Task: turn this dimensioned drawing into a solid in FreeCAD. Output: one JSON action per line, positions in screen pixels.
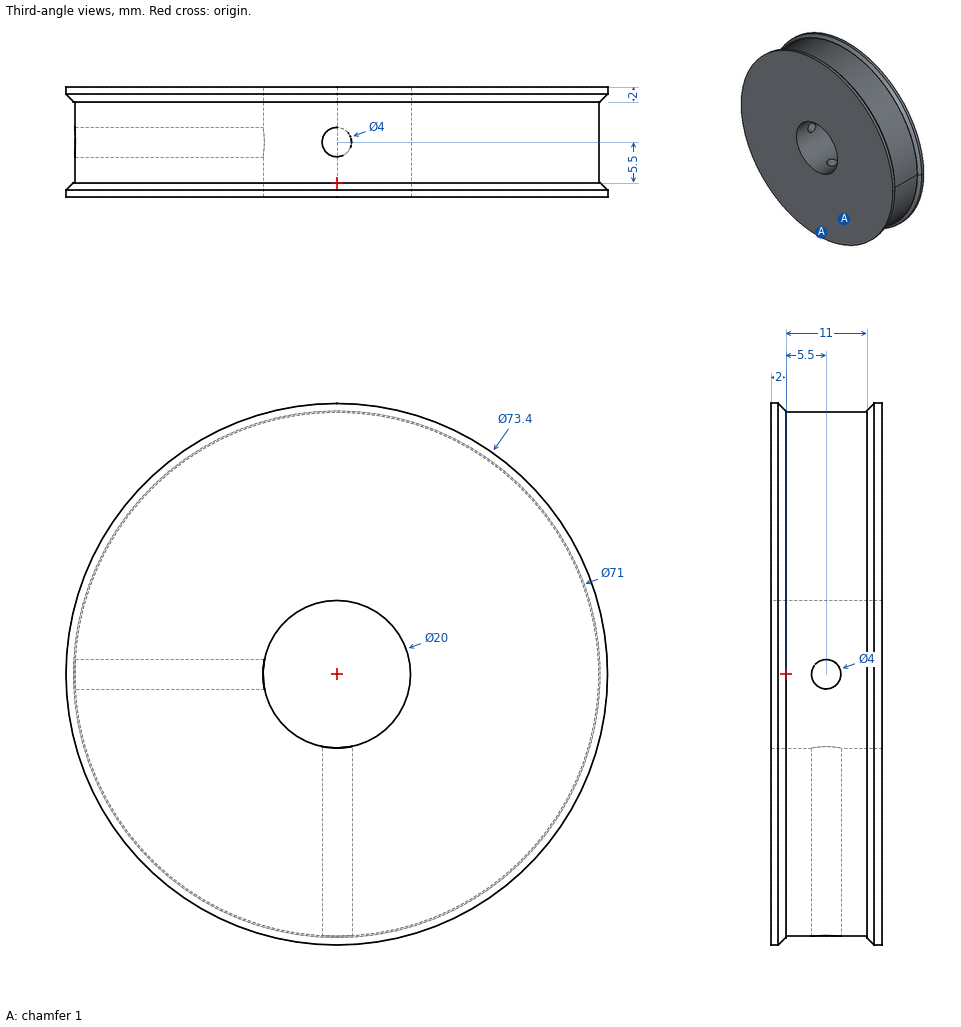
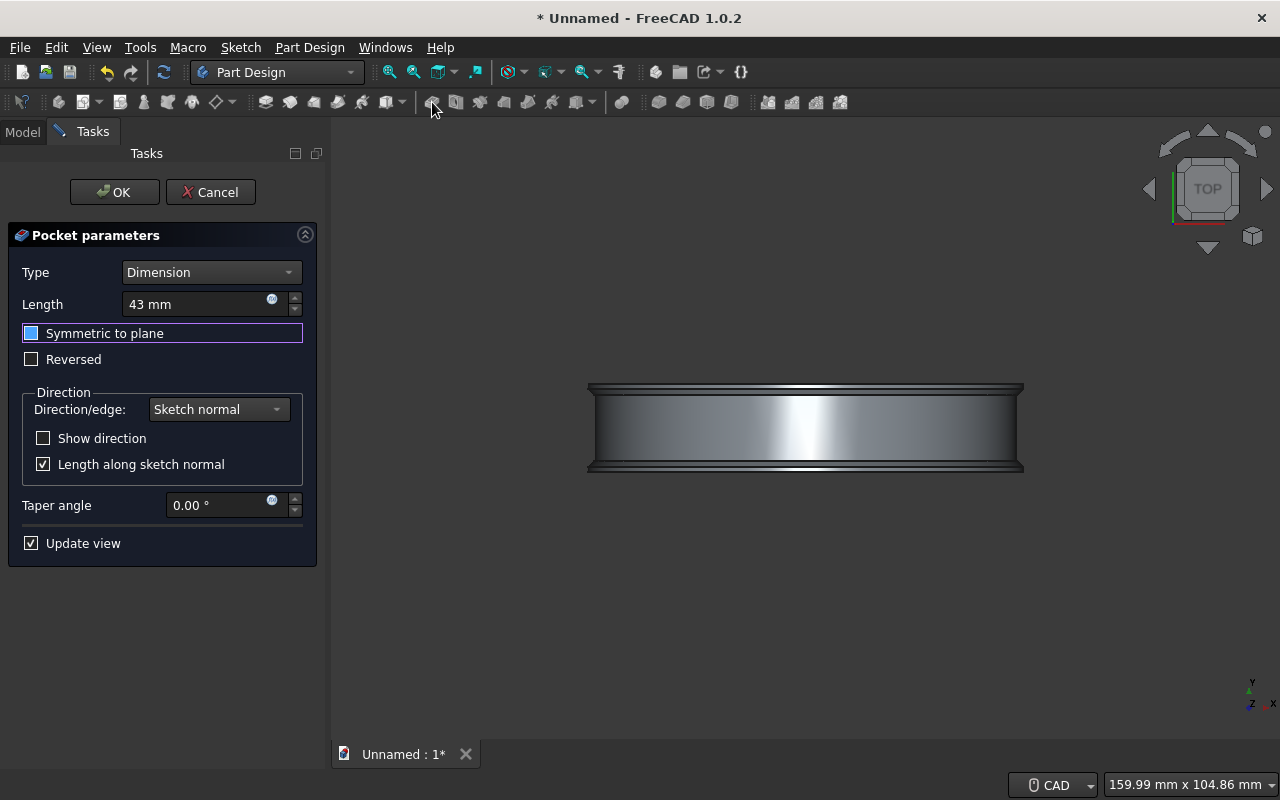
{"action": "left_click", "coordinate": [115, 192]}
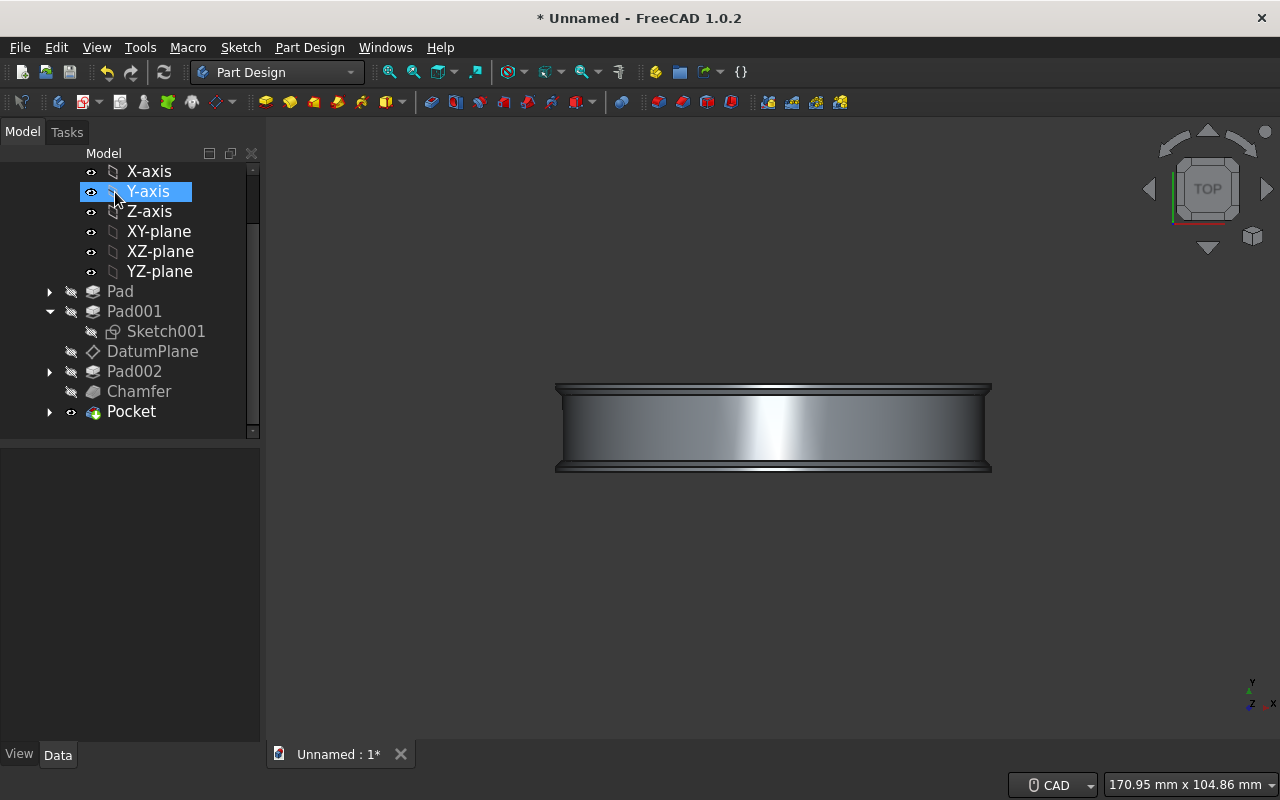
{"action": "left_click", "coordinate": [390, 72]}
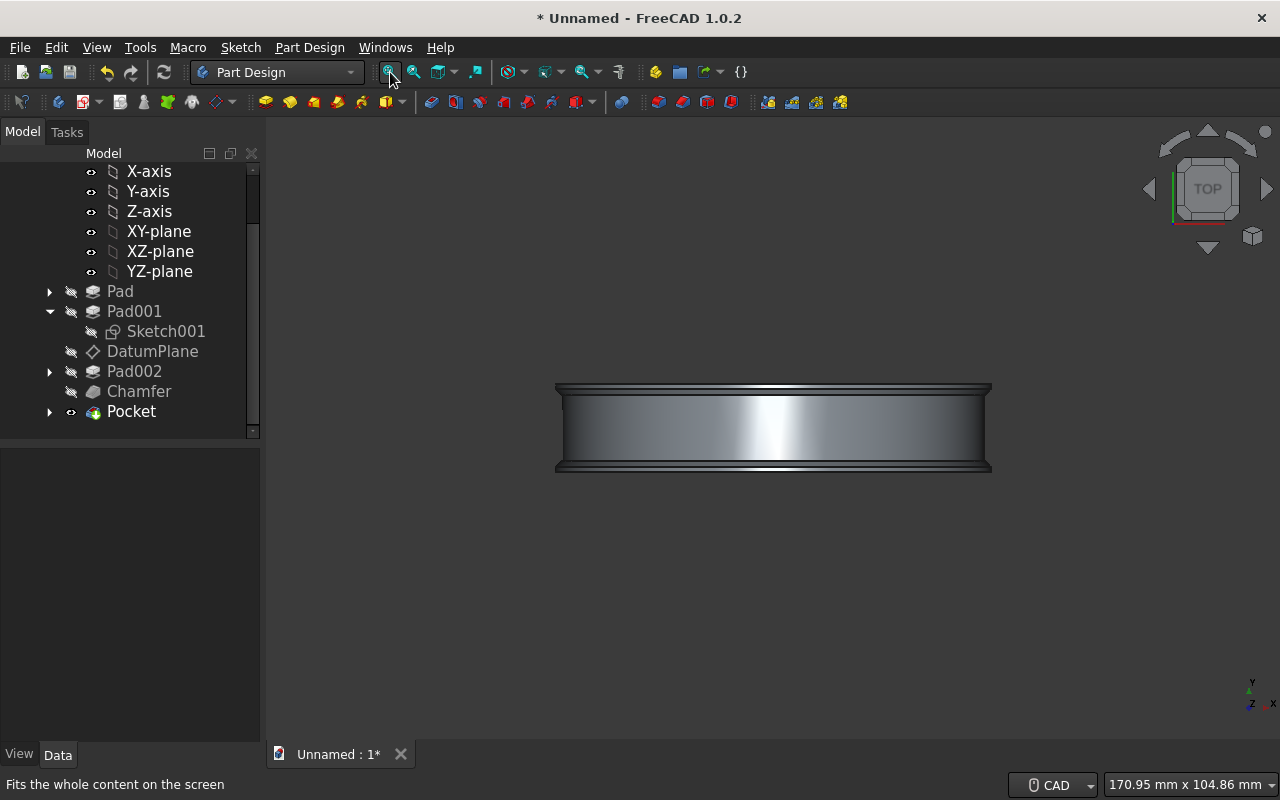
{"action": "left_click", "coordinate": [84, 102]}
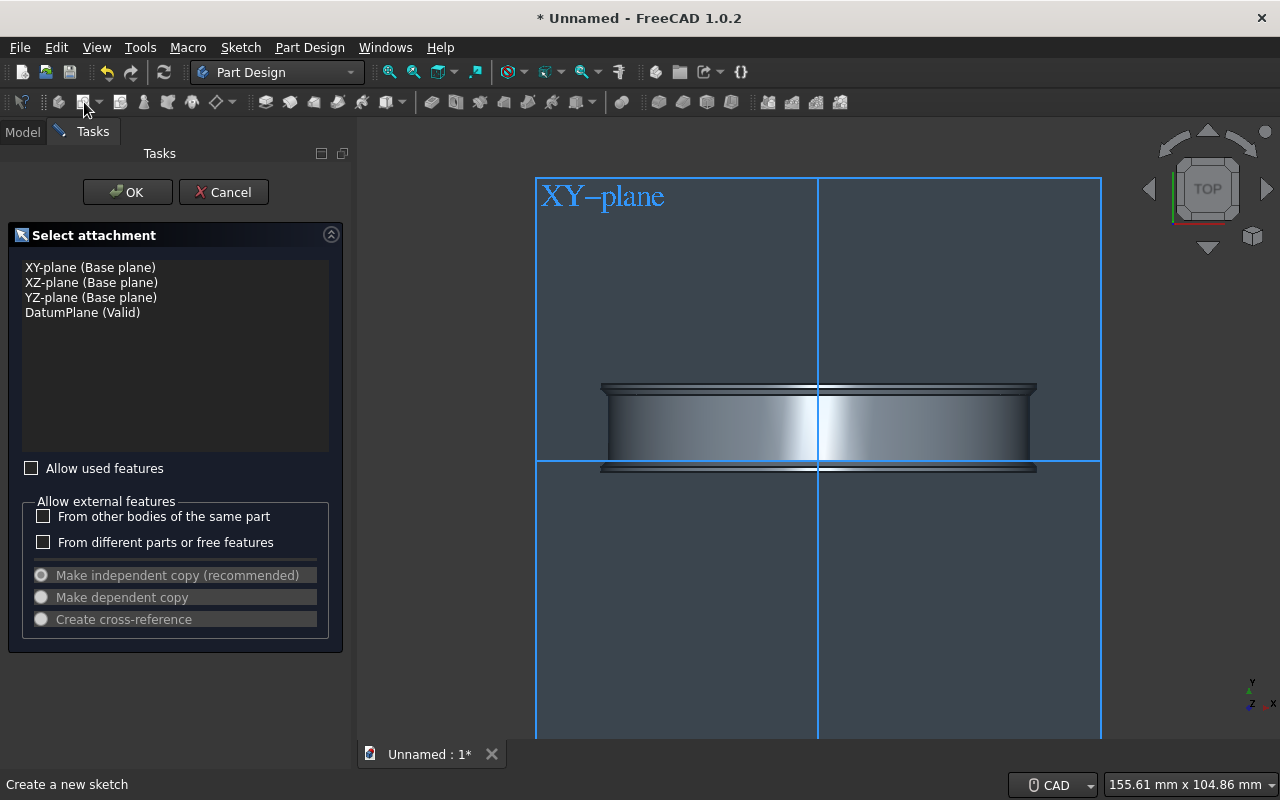
{"action": "left_click", "coordinate": [82, 298]}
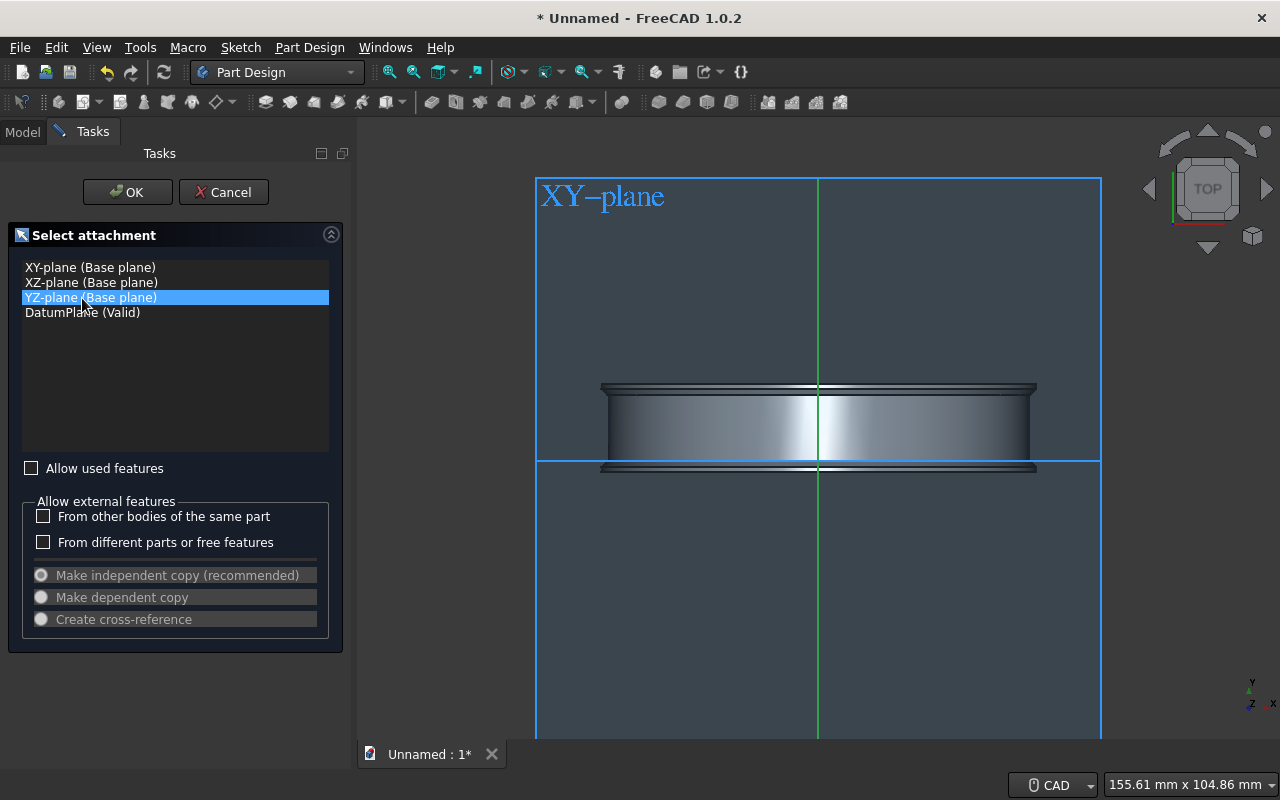
{"action": "left_click", "coordinate": [128, 192]}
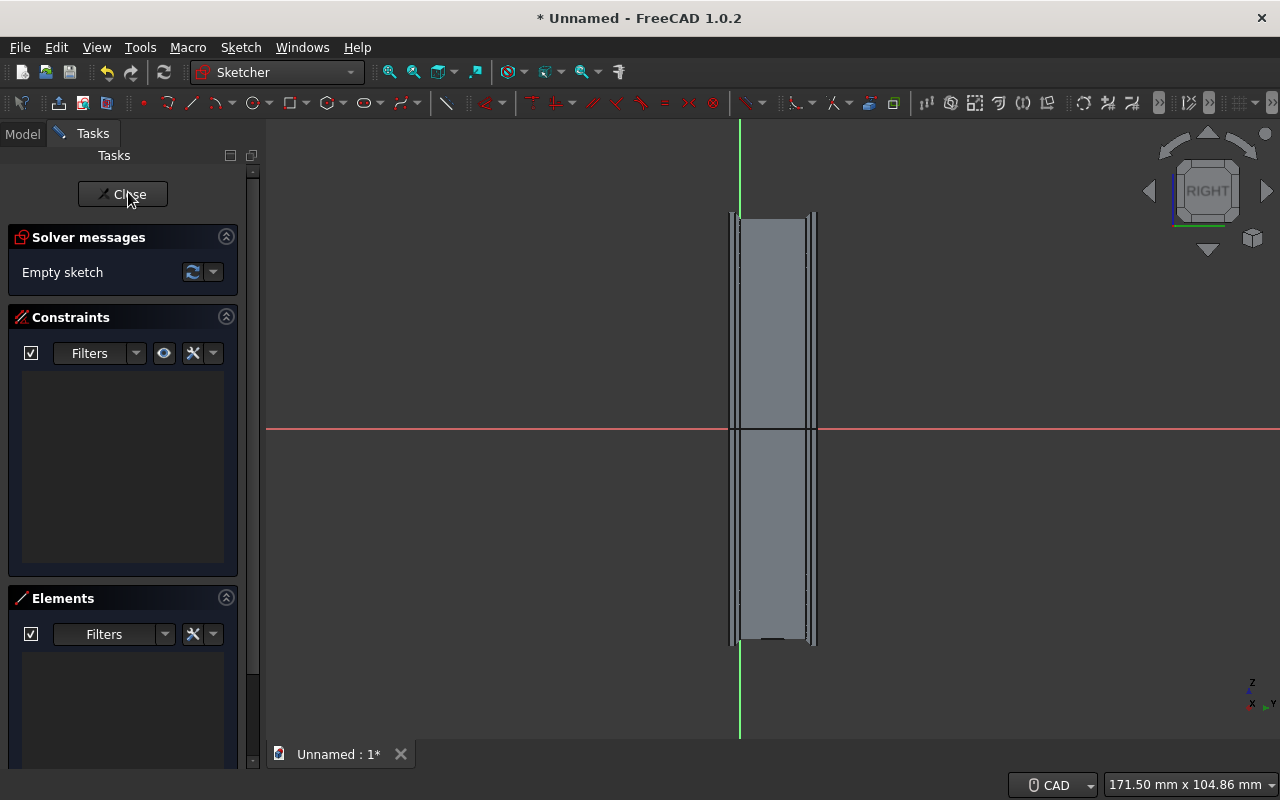
{"action": "left_click", "coordinate": [108, 104]}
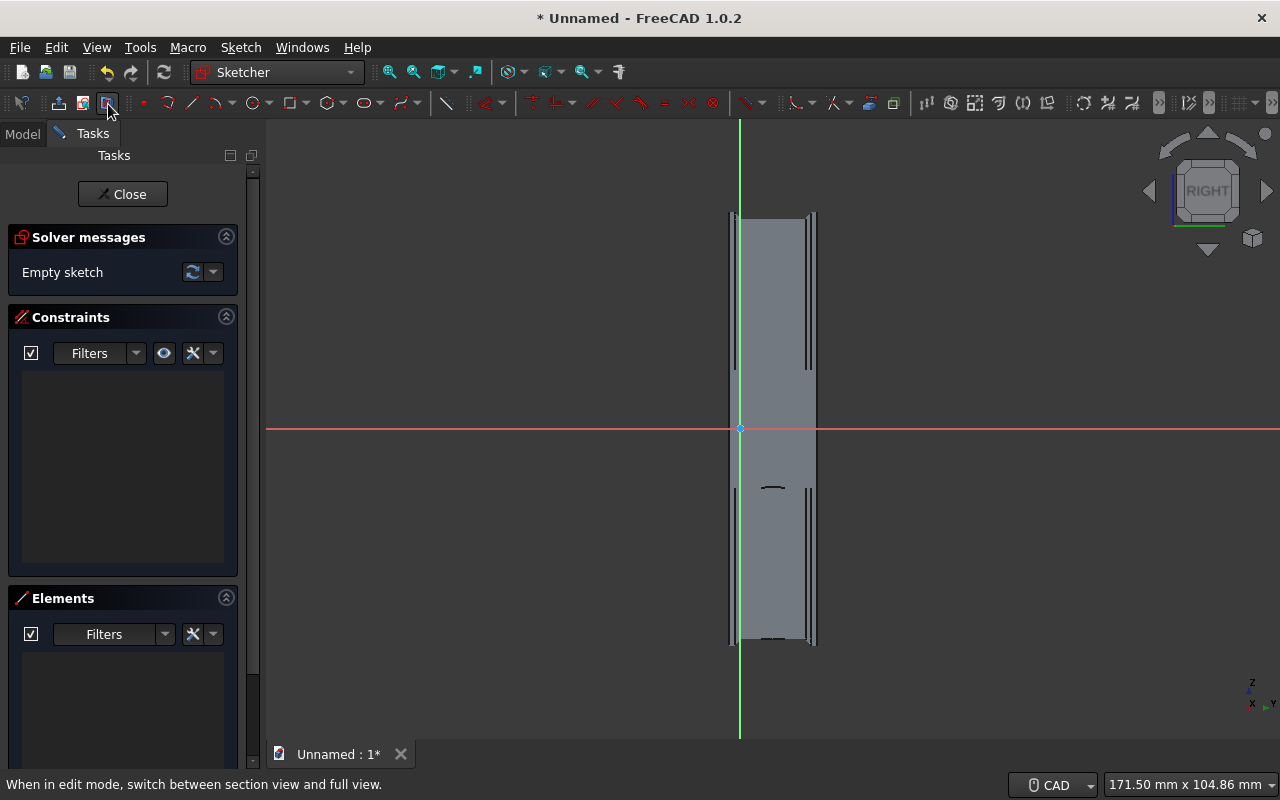
{"action": "scroll", "coordinate": [767, 429], "scroll_direction": "up", "scroll_amount": 13}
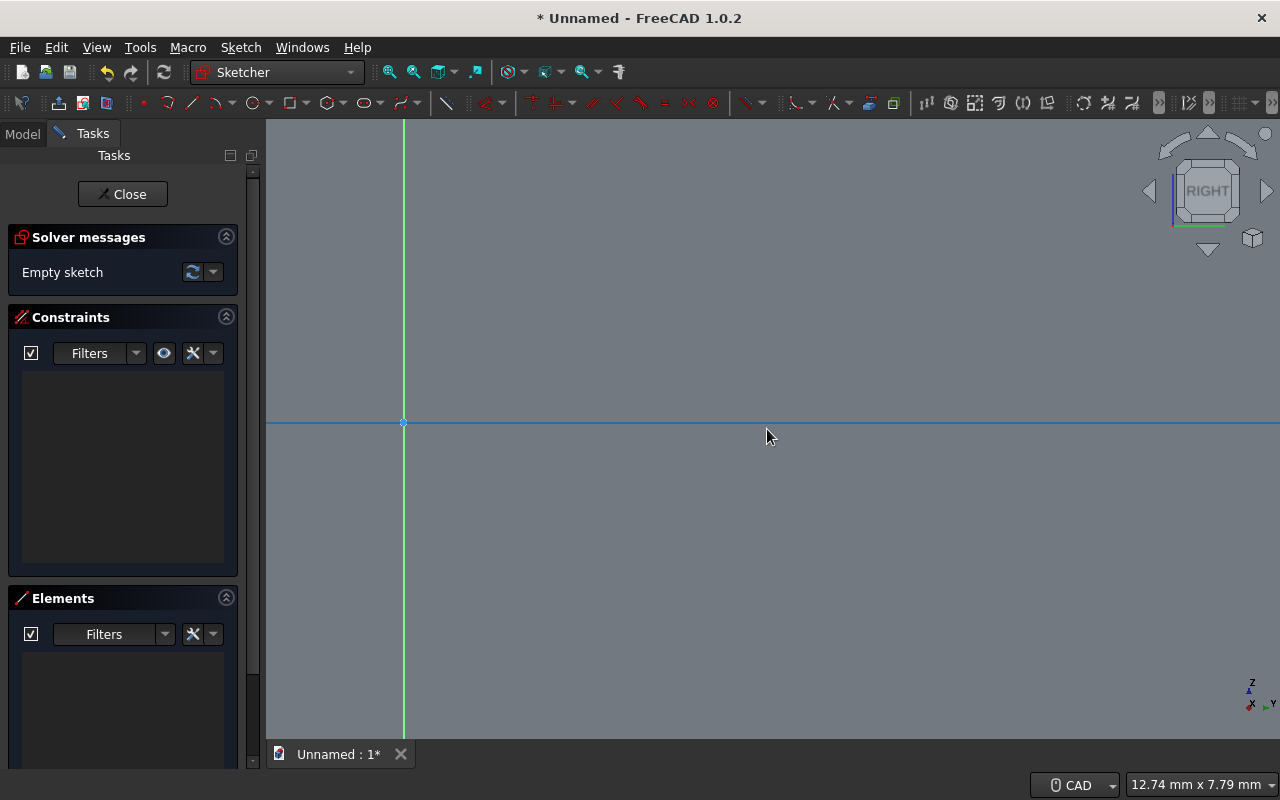
{"action": "left_click", "coordinate": [254, 104]}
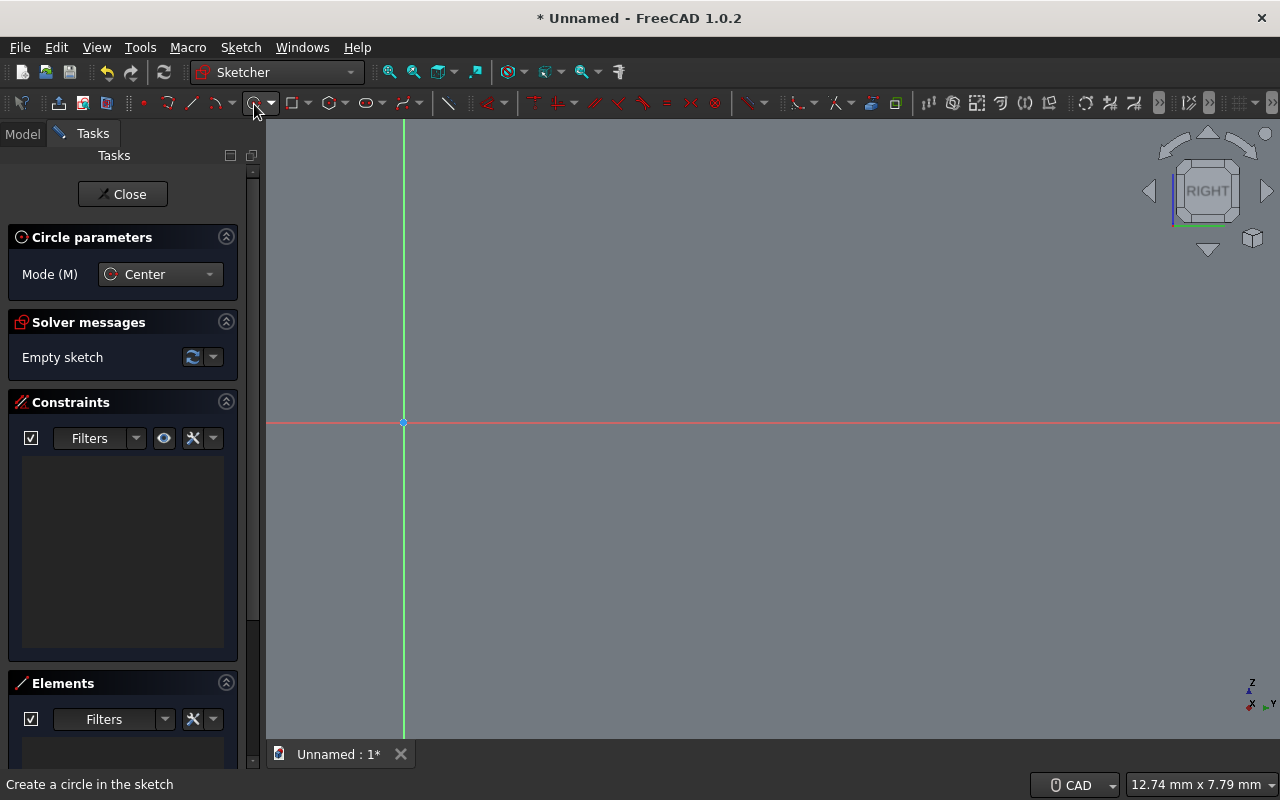
{"action": "left_click", "coordinate": [842, 423]}
{"action": "left_click", "coordinate": [954, 310]}
{"action": "key", "text": "Escape"}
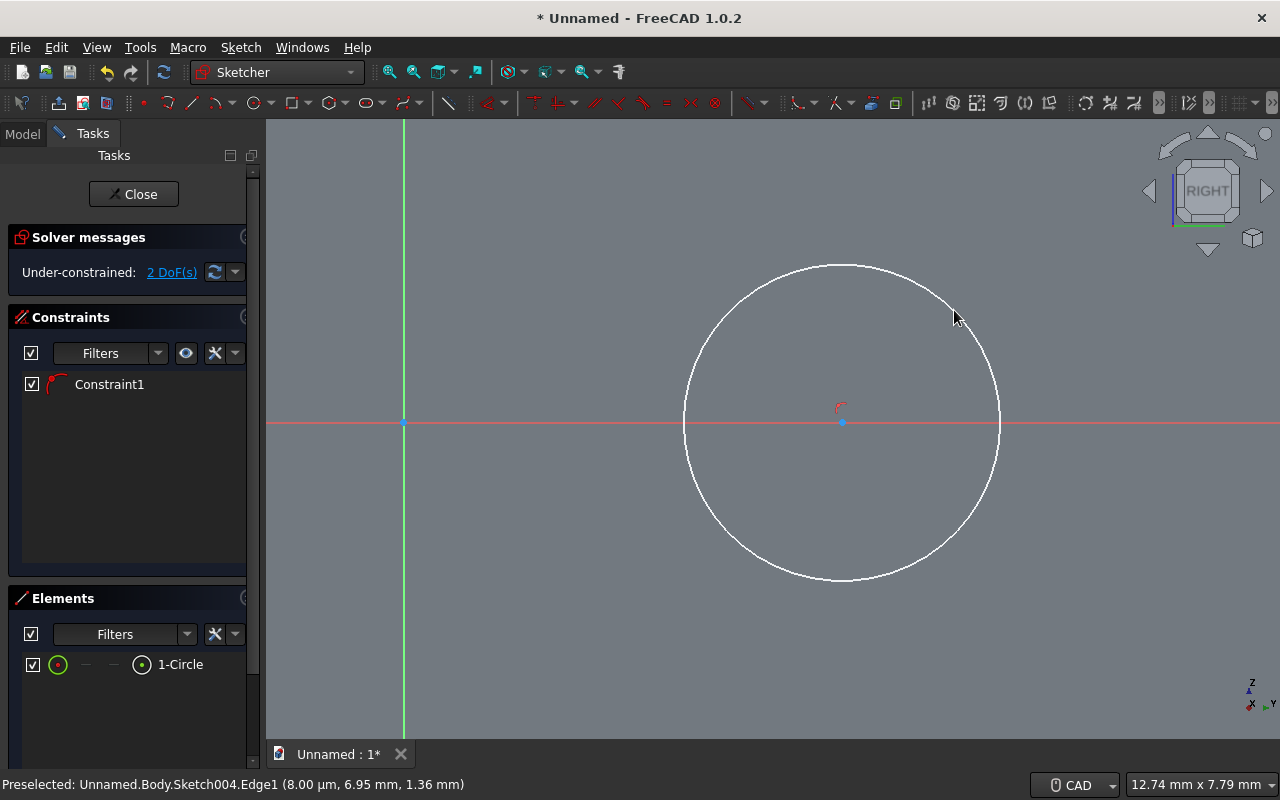
{"action": "left_click", "coordinate": [488, 104]}